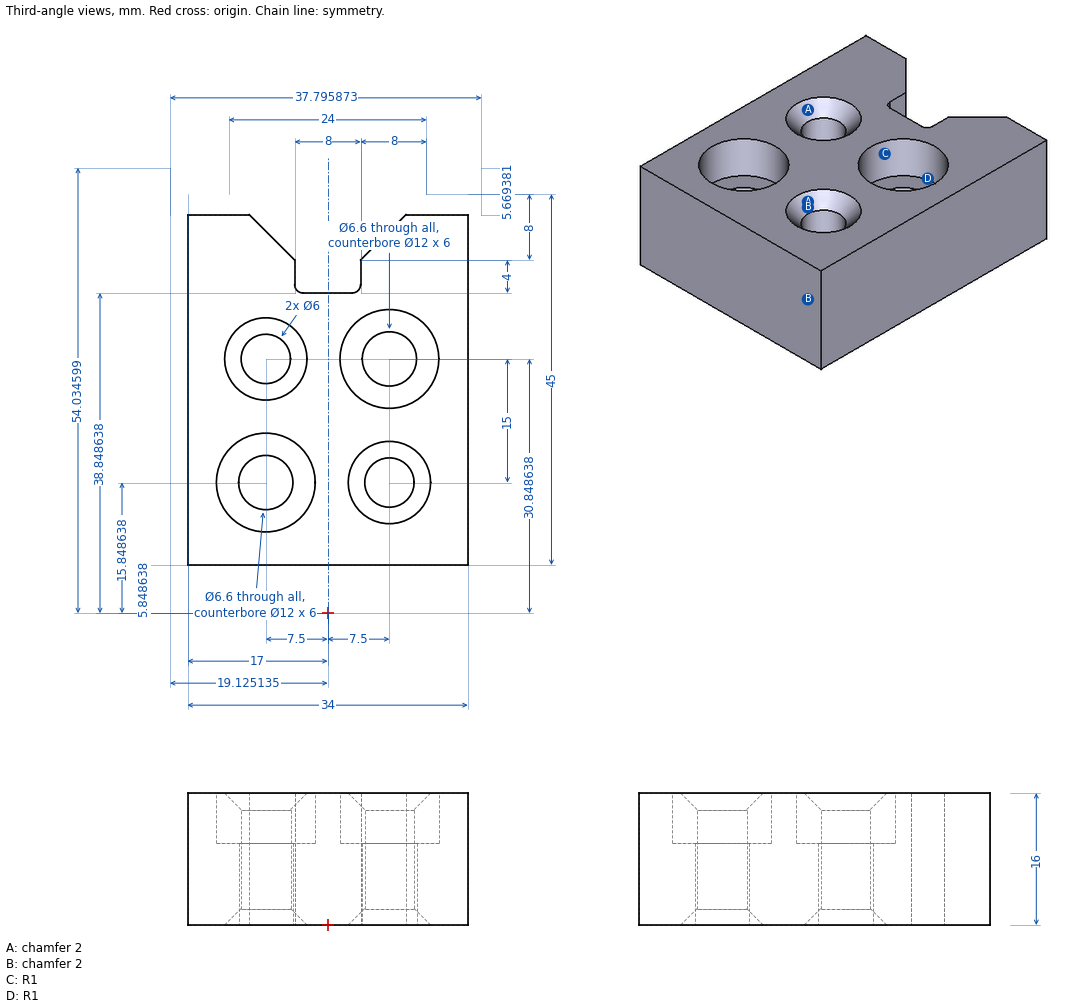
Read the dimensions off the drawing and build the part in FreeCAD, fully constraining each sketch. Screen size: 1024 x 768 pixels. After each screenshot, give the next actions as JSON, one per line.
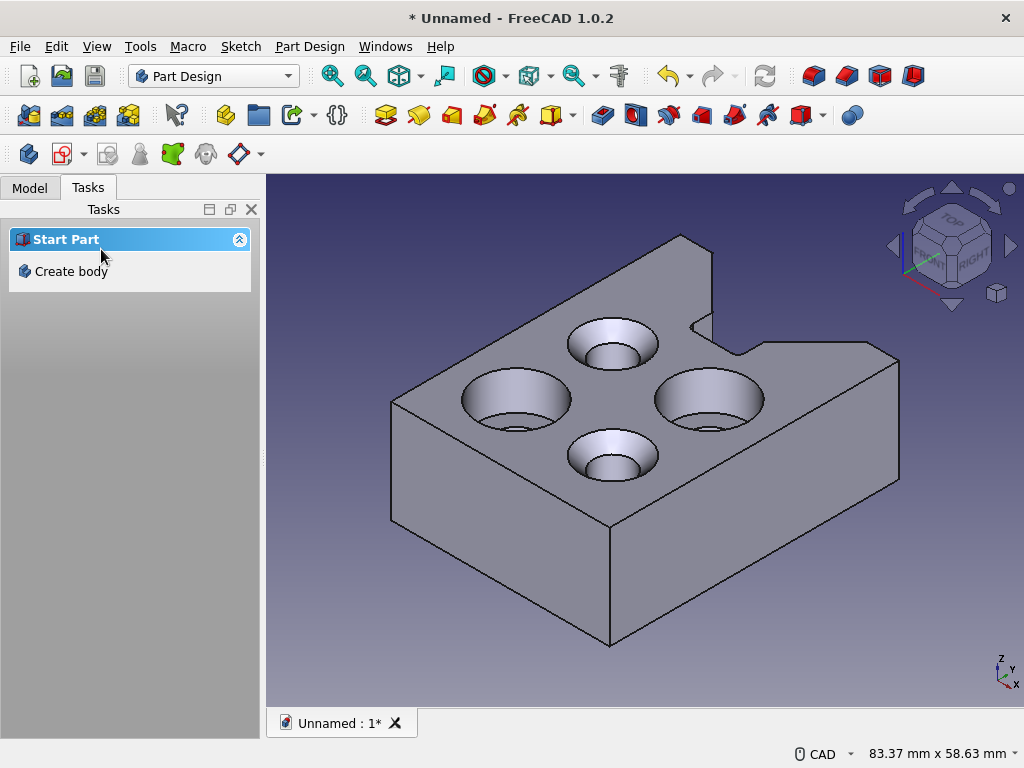
{"action": "left_click", "coordinate": [665, 296]}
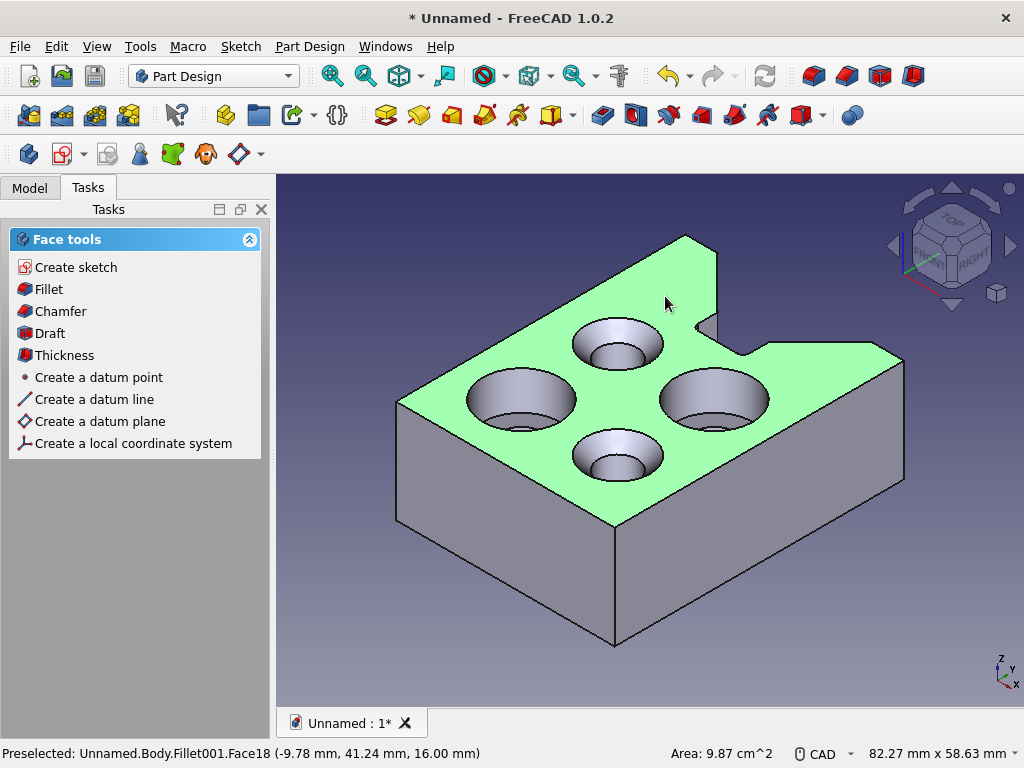
{"action": "left_click", "coordinate": [62, 154]}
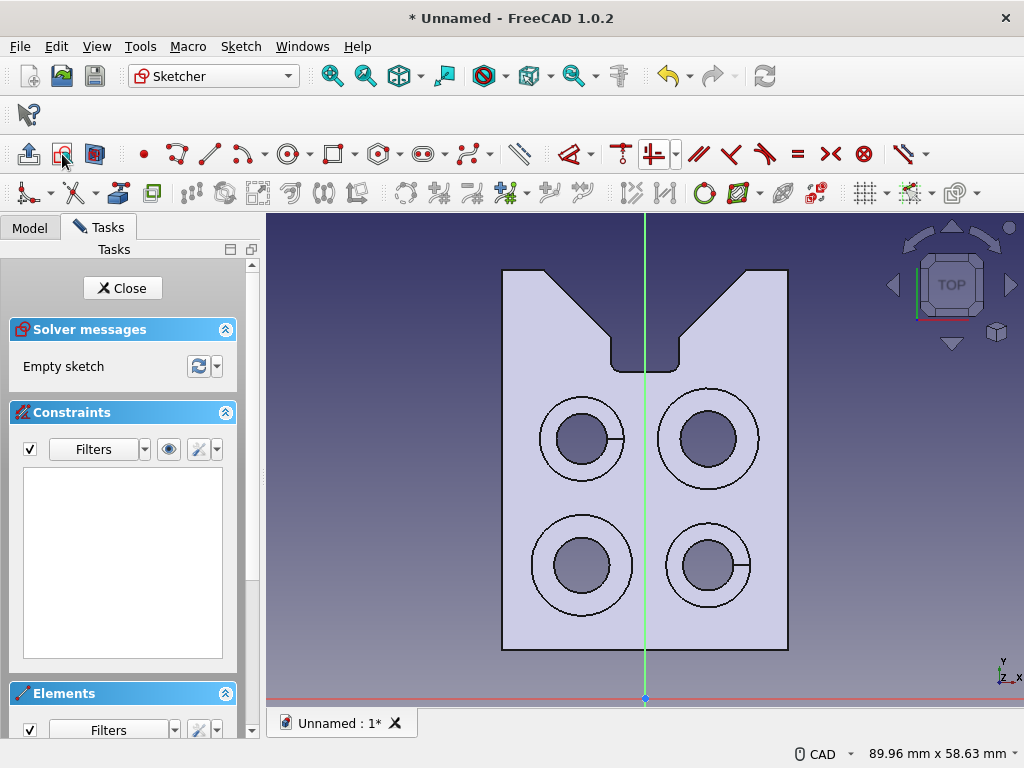
{"action": "scroll", "coordinate": [441, 437], "scroll_direction": "down", "scroll_amount": 2}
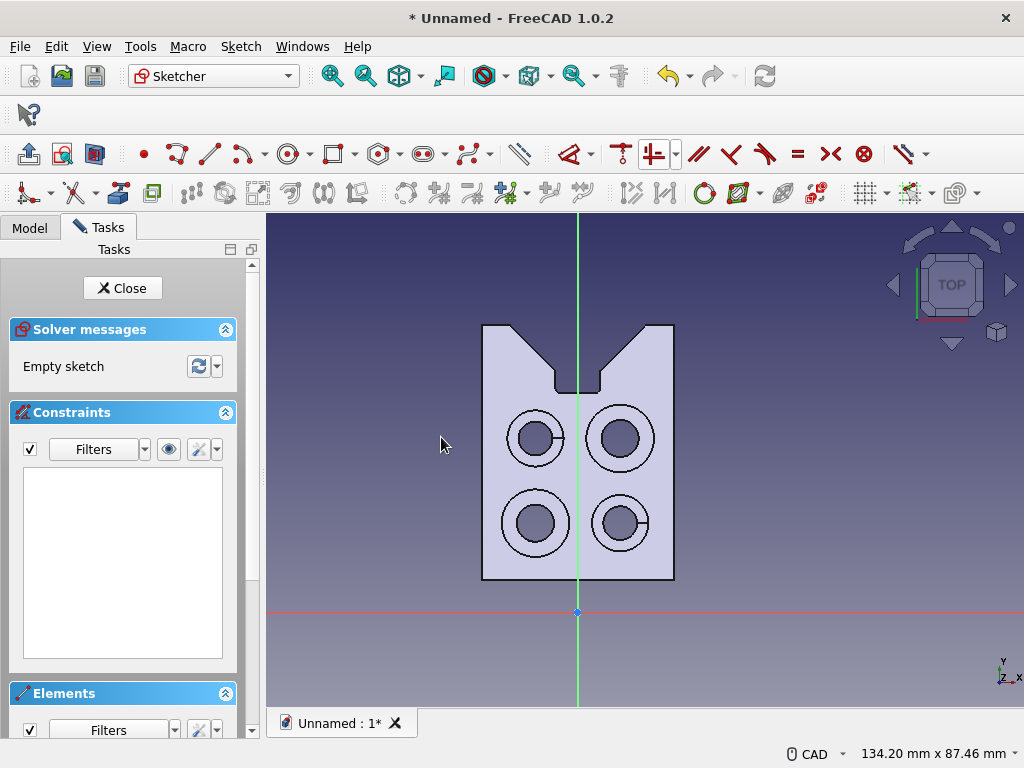
{"action": "left_click", "coordinate": [332, 154]}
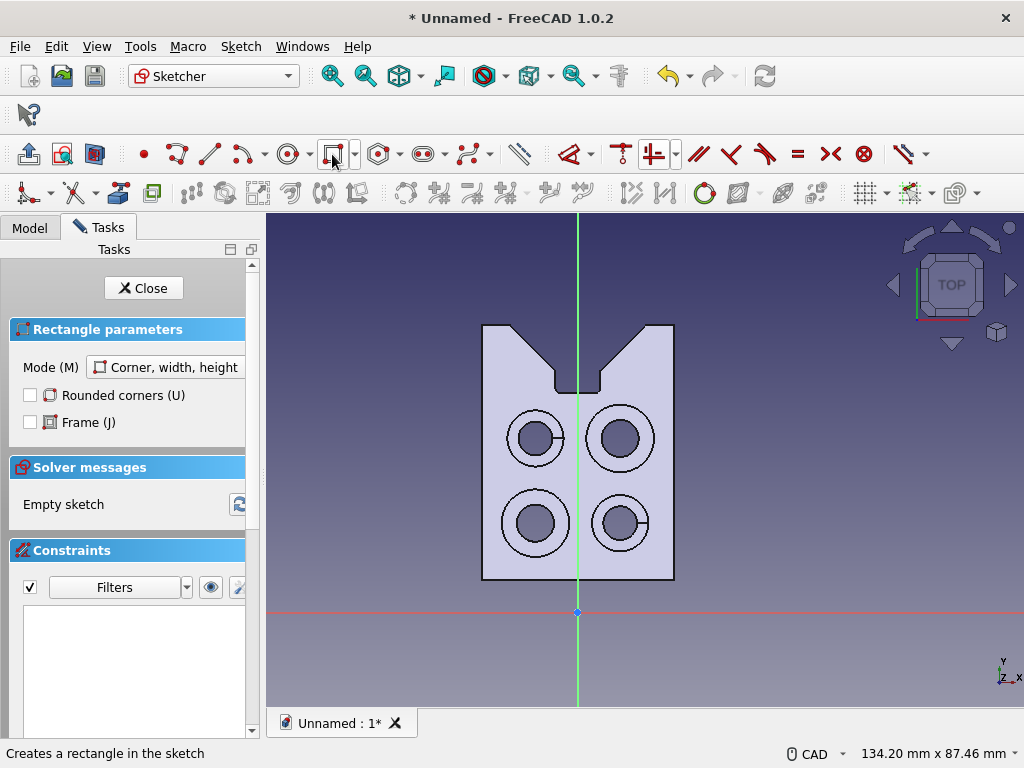
{"action": "left_click", "coordinate": [470, 307]}
{"action": "mouse_move", "coordinate": [683, 340]}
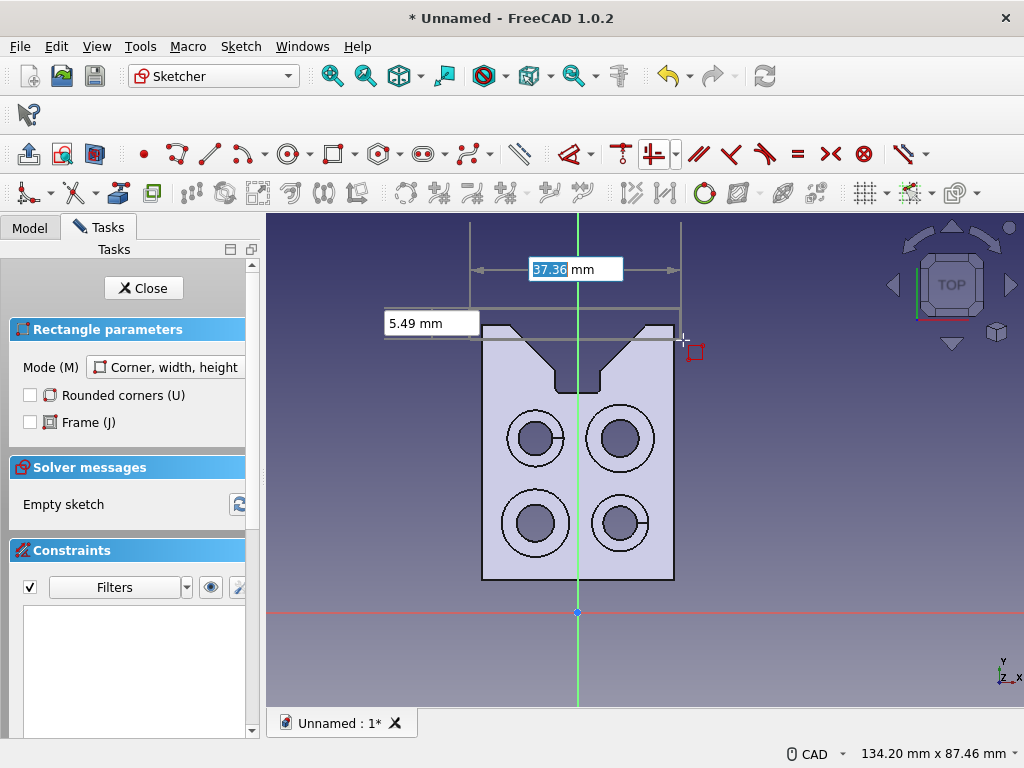
{"action": "type", "text": "37.795873"}
{"action": "key", "text": "Tab"}
{"action": "type", "text": "5.669381"}
{"action": "key", "text": "Return"}
{"action": "key", "text": "Escape"}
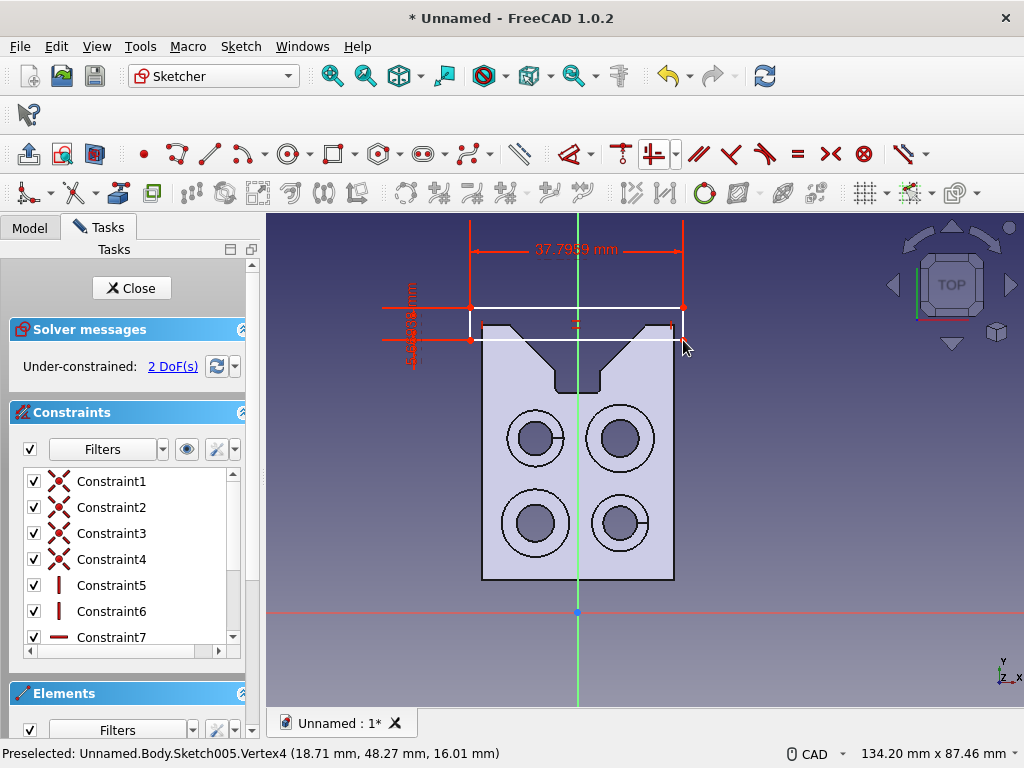
{"action": "left_click", "coordinate": [568, 154]}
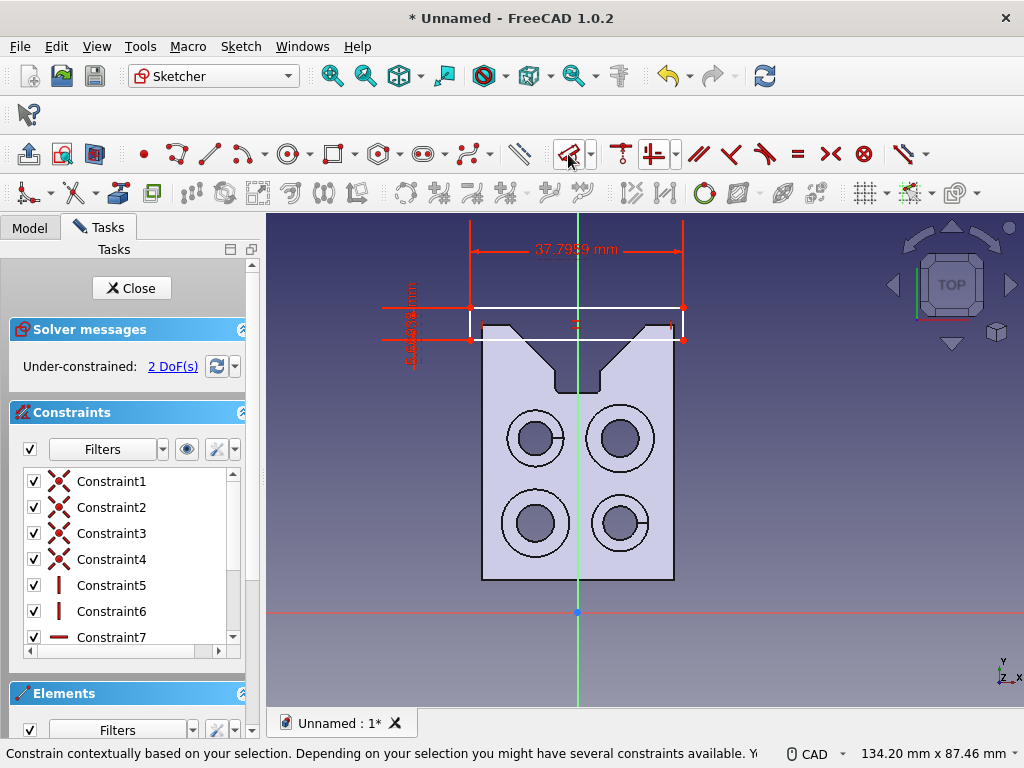
{"action": "left_click", "coordinate": [470, 308]}
{"action": "left_click", "coordinate": [524, 647]}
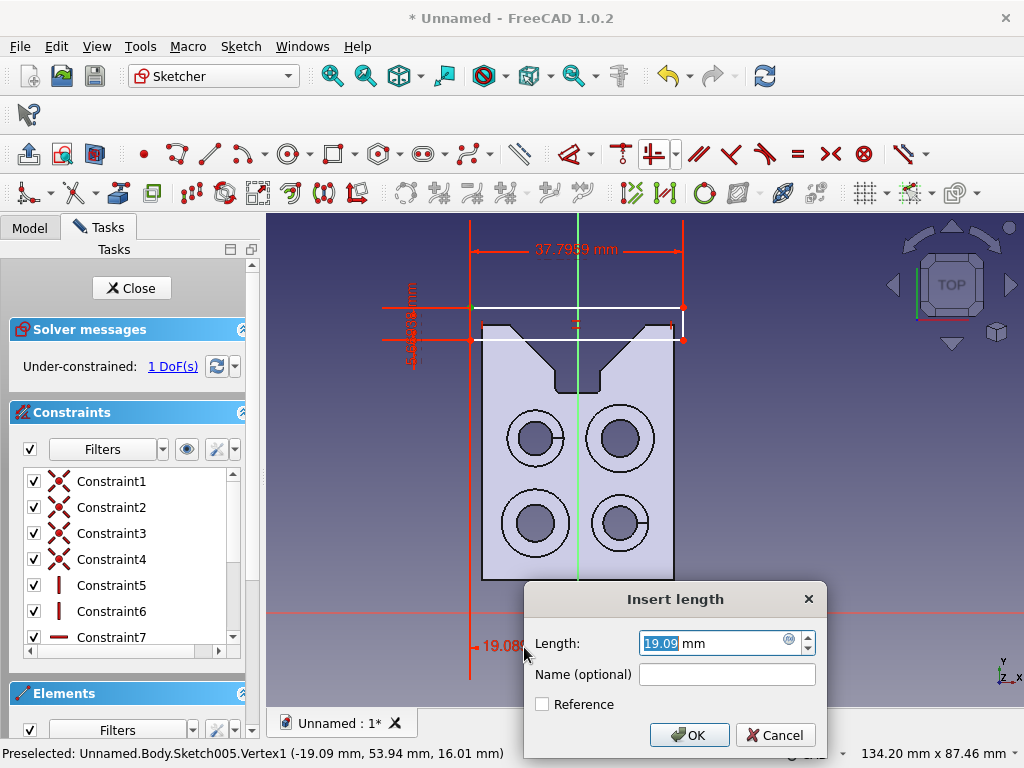
{"action": "type", "text": "19.125135"}
{"action": "key", "text": "Return"}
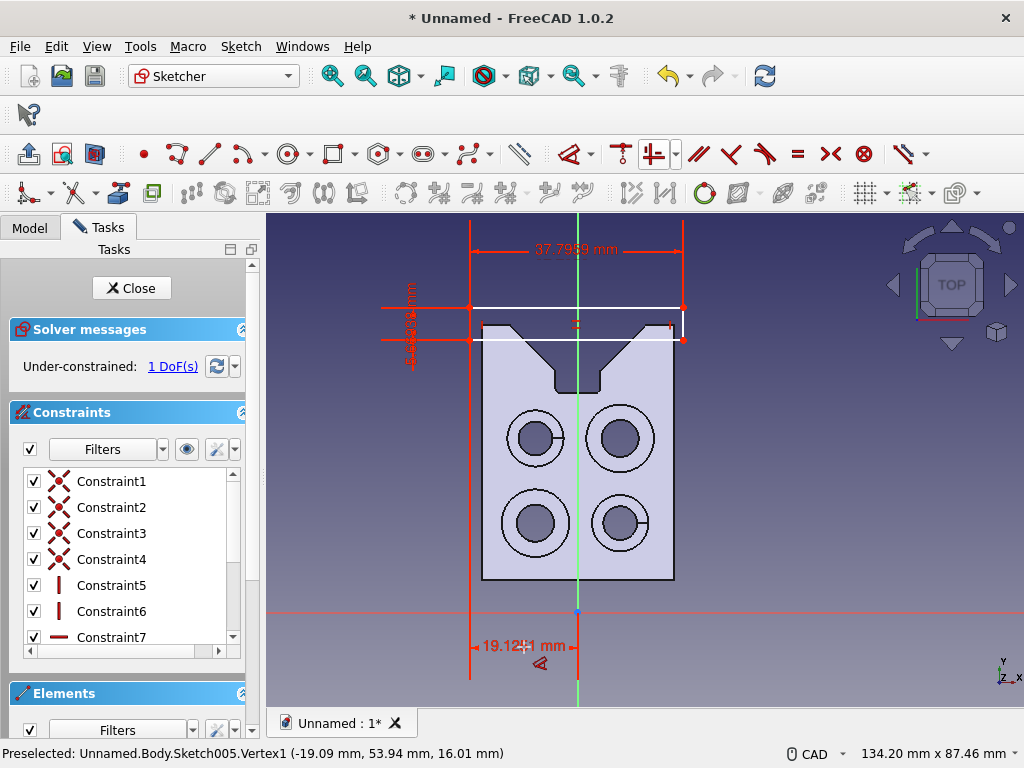
{"action": "left_click", "coordinate": [470, 308]}
{"action": "left_click", "coordinate": [436, 460]}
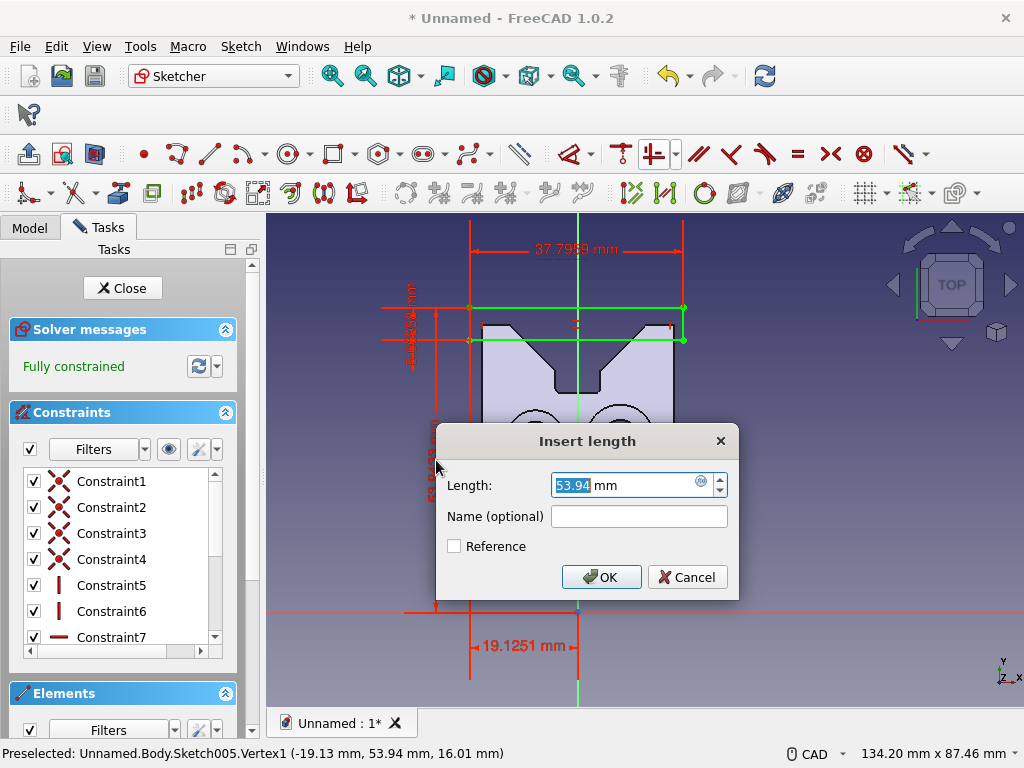
{"action": "type", "text": "54.034599"}
{"action": "key", "text": "Return"}
{"action": "key", "text": "Escape"}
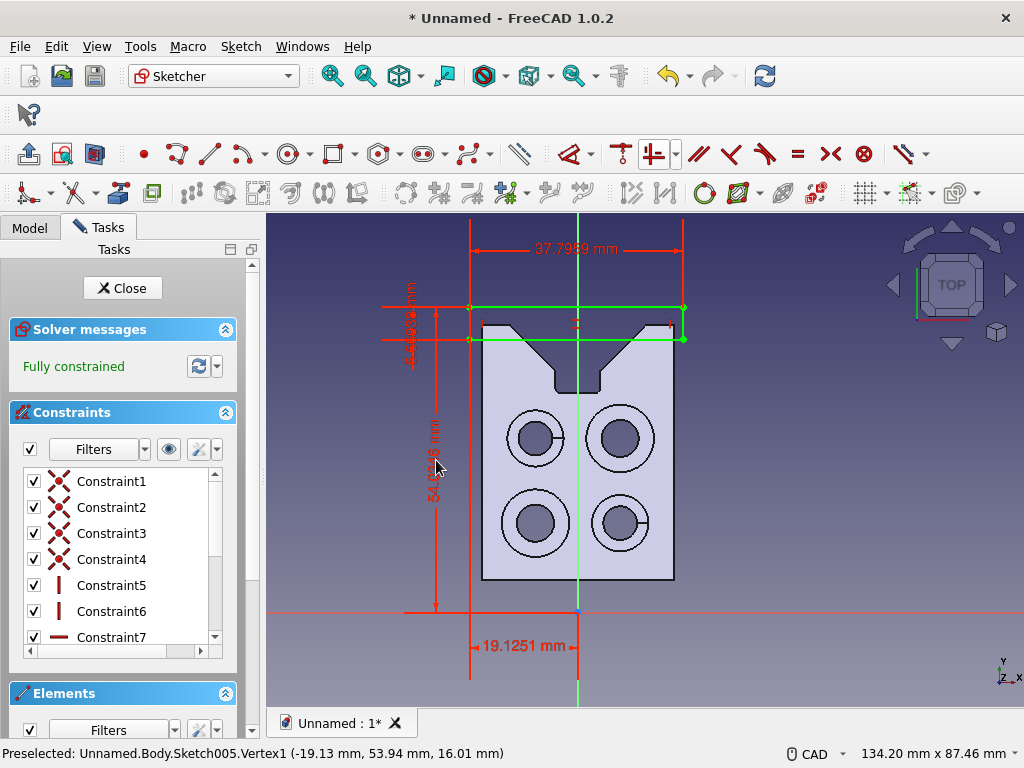
{"action": "left_click", "coordinate": [123, 288]}